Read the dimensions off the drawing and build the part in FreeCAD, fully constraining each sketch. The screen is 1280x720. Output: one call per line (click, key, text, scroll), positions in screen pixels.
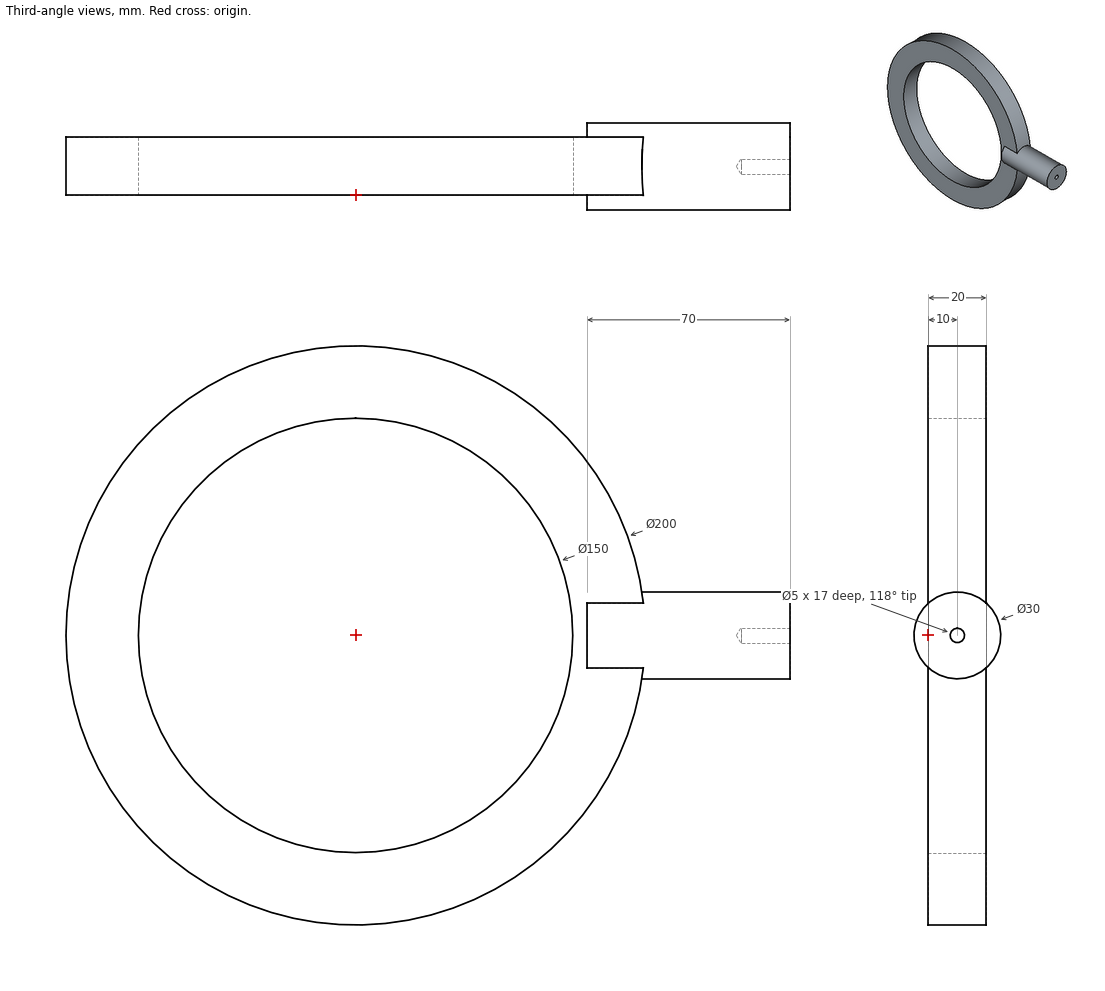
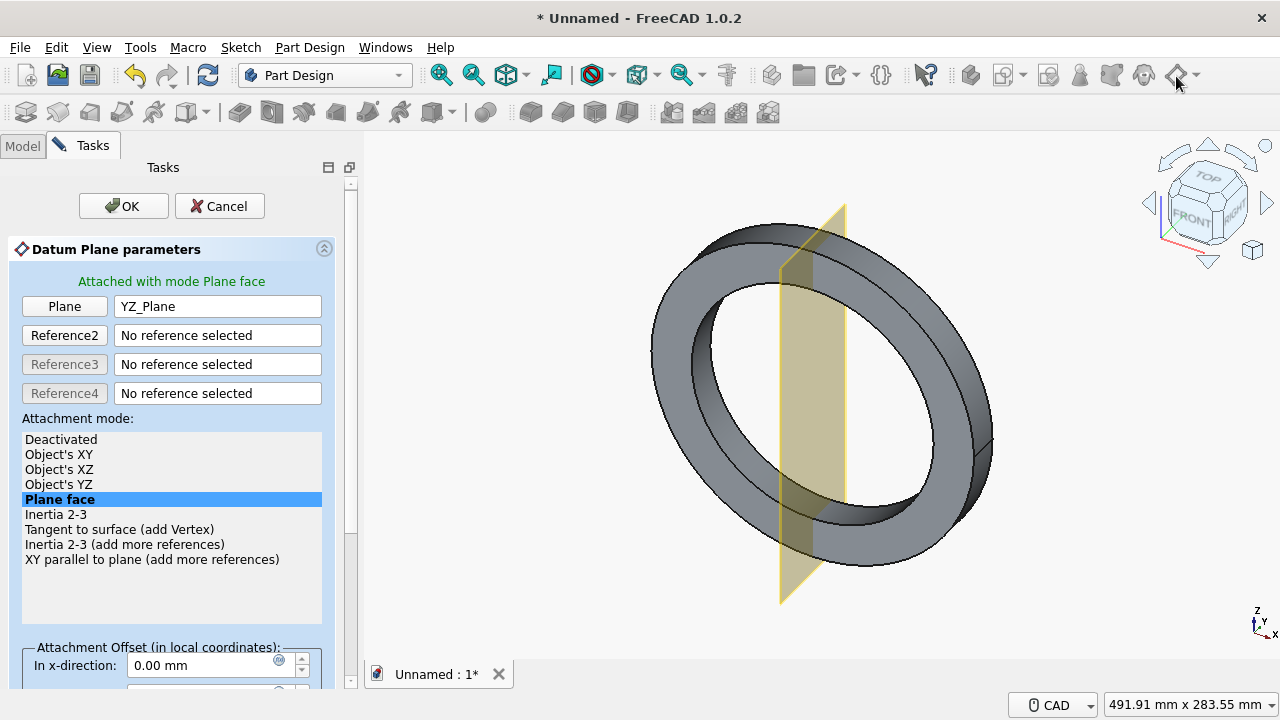
scroll(351, 432, down, 2)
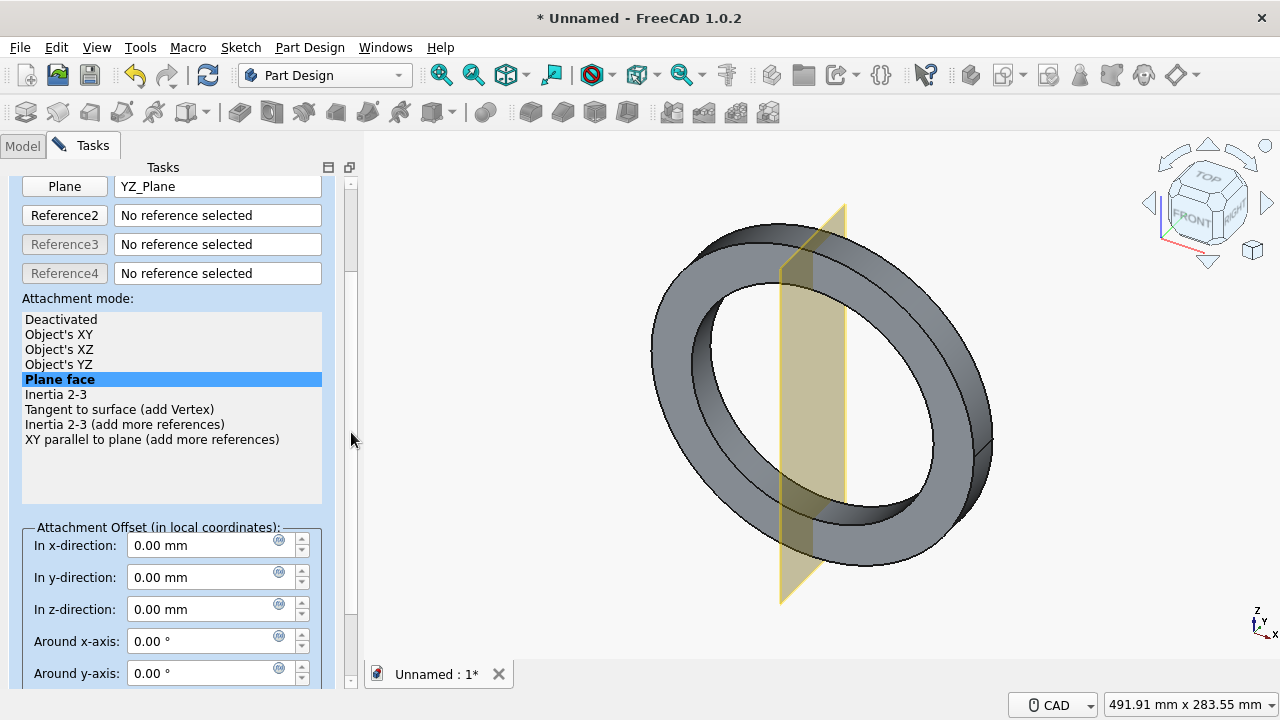
triple_click(210, 609)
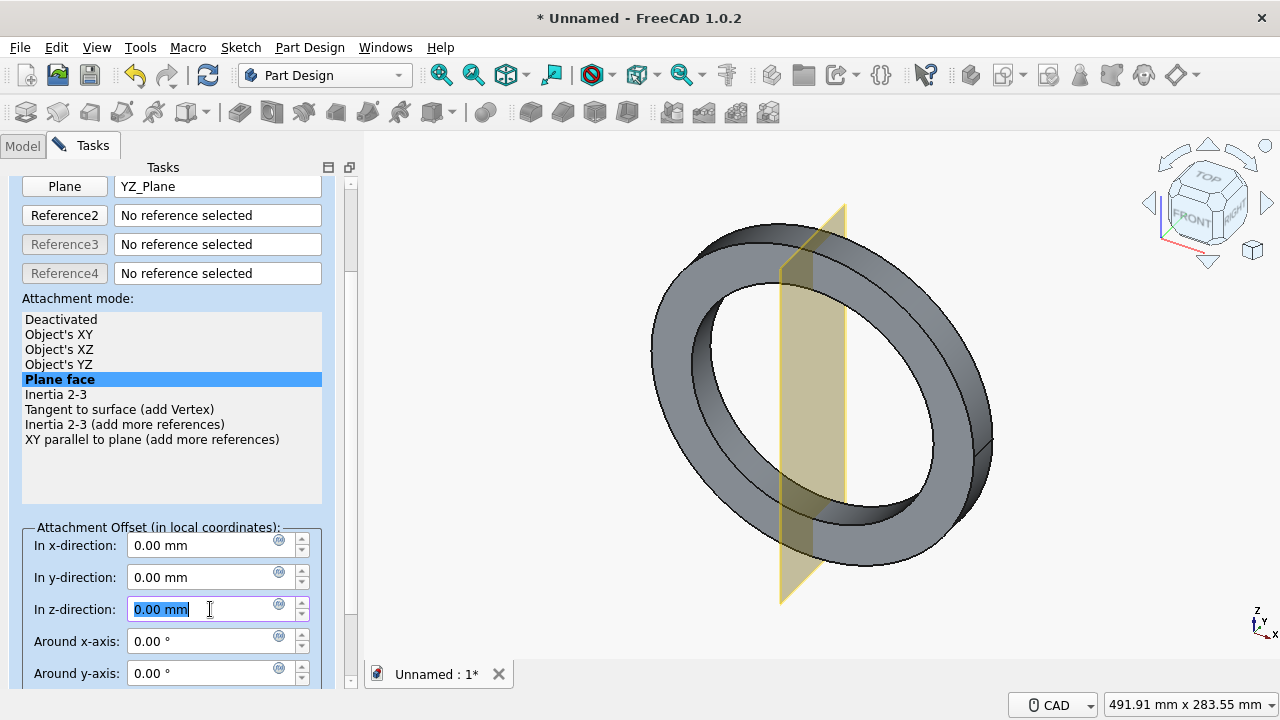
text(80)
key(Tab)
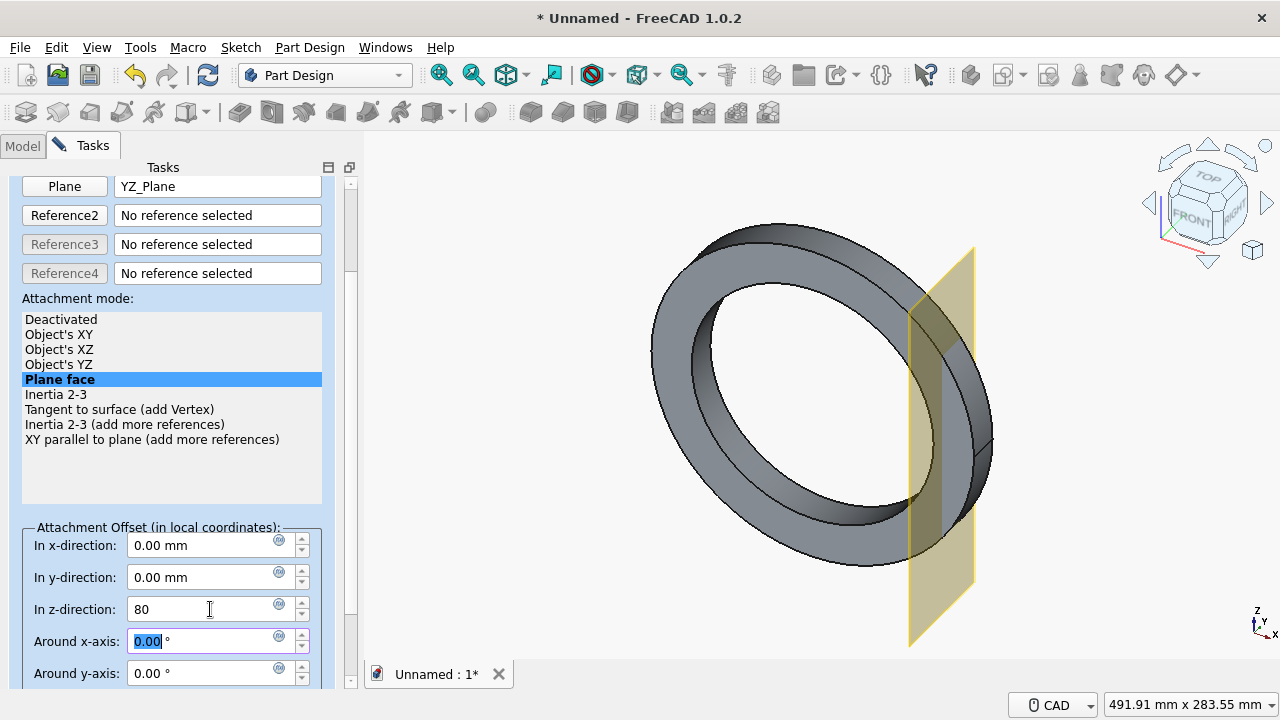
scroll(351, 432, up, 3)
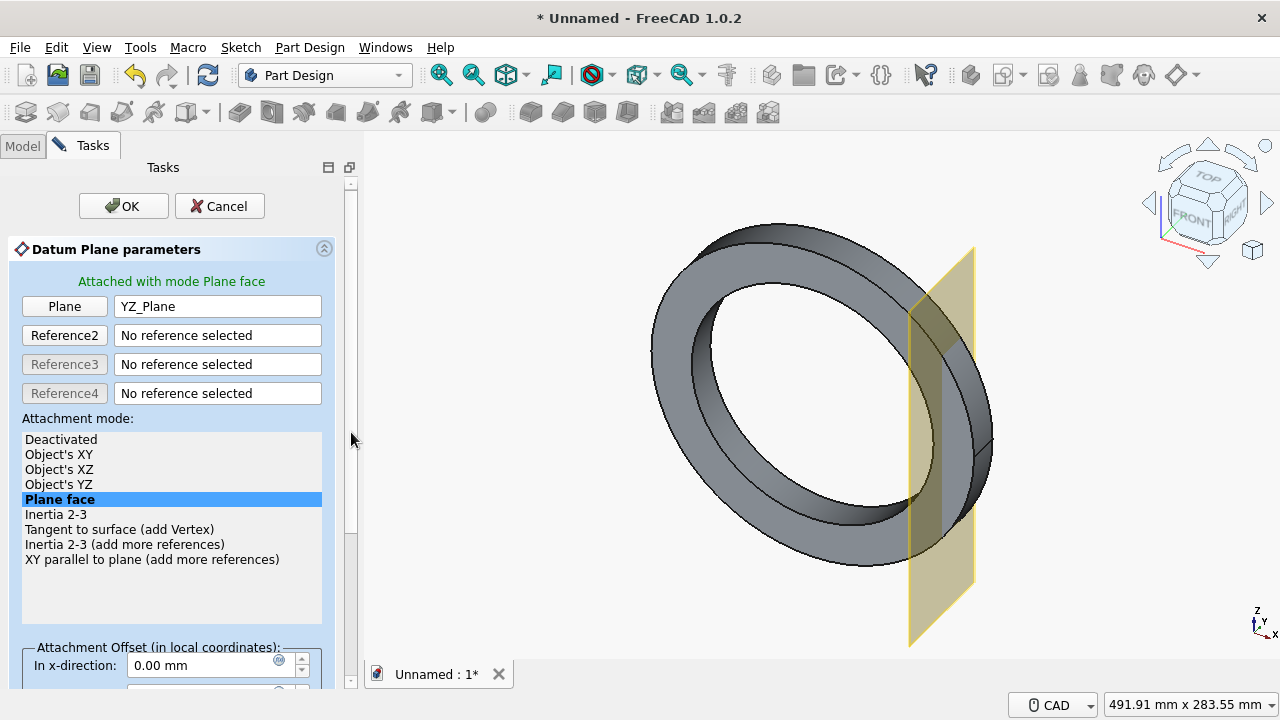
click(124, 206)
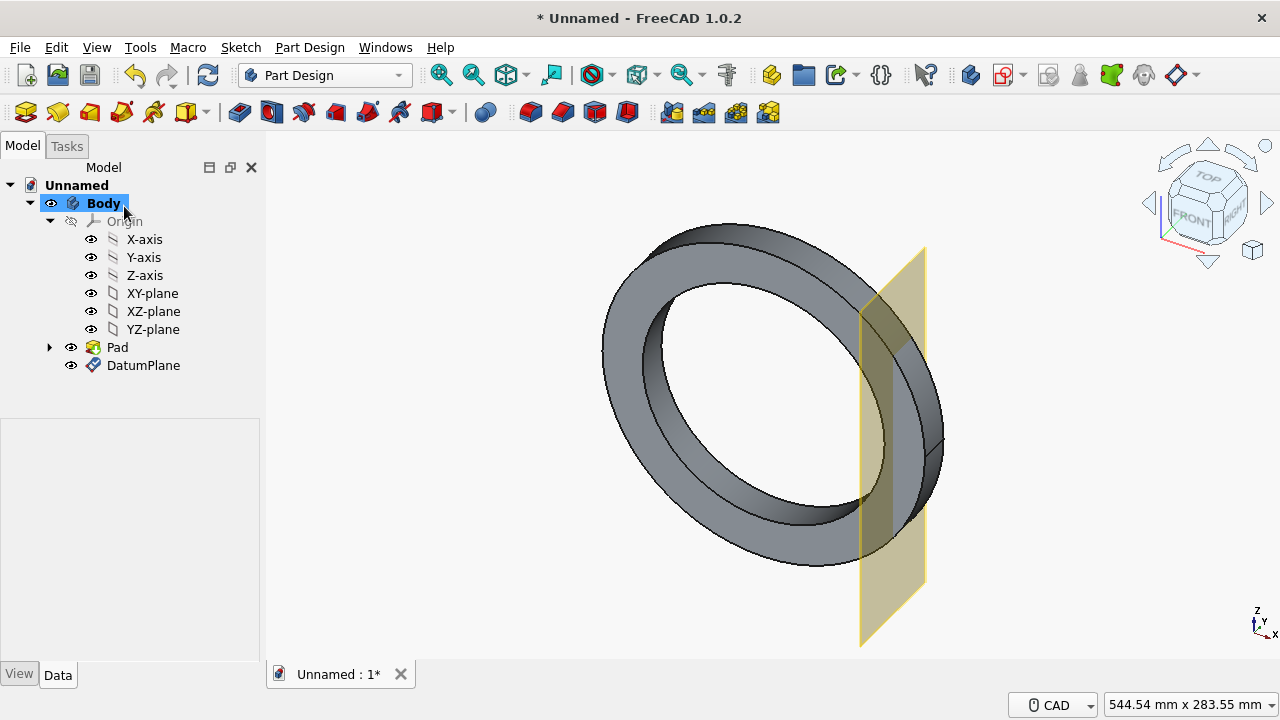
click(116, 365)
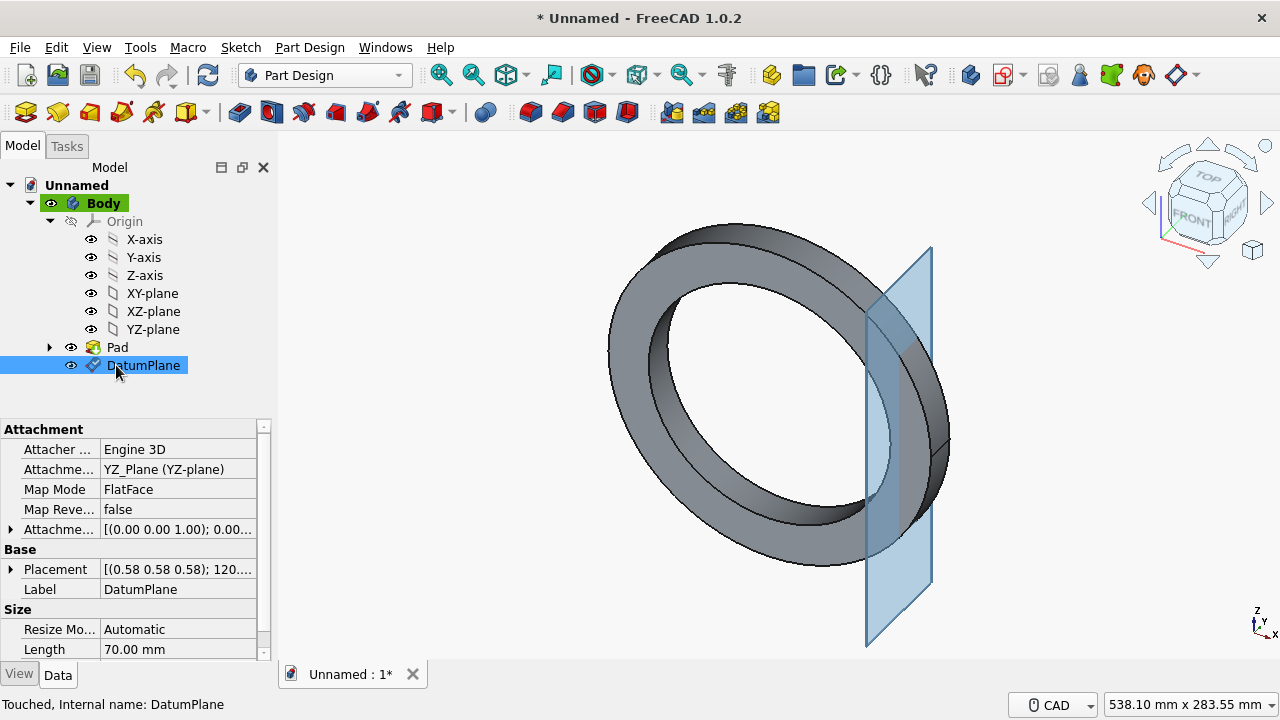
click(1004, 76)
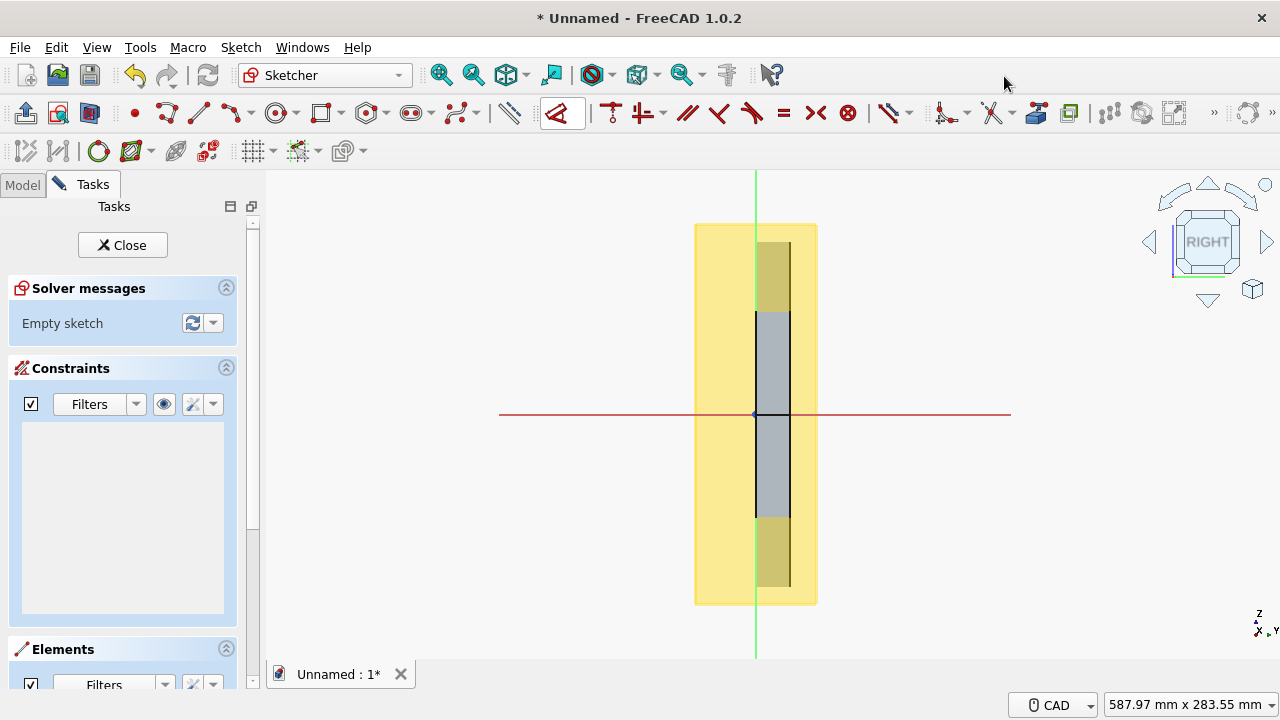
key(q)
key(s)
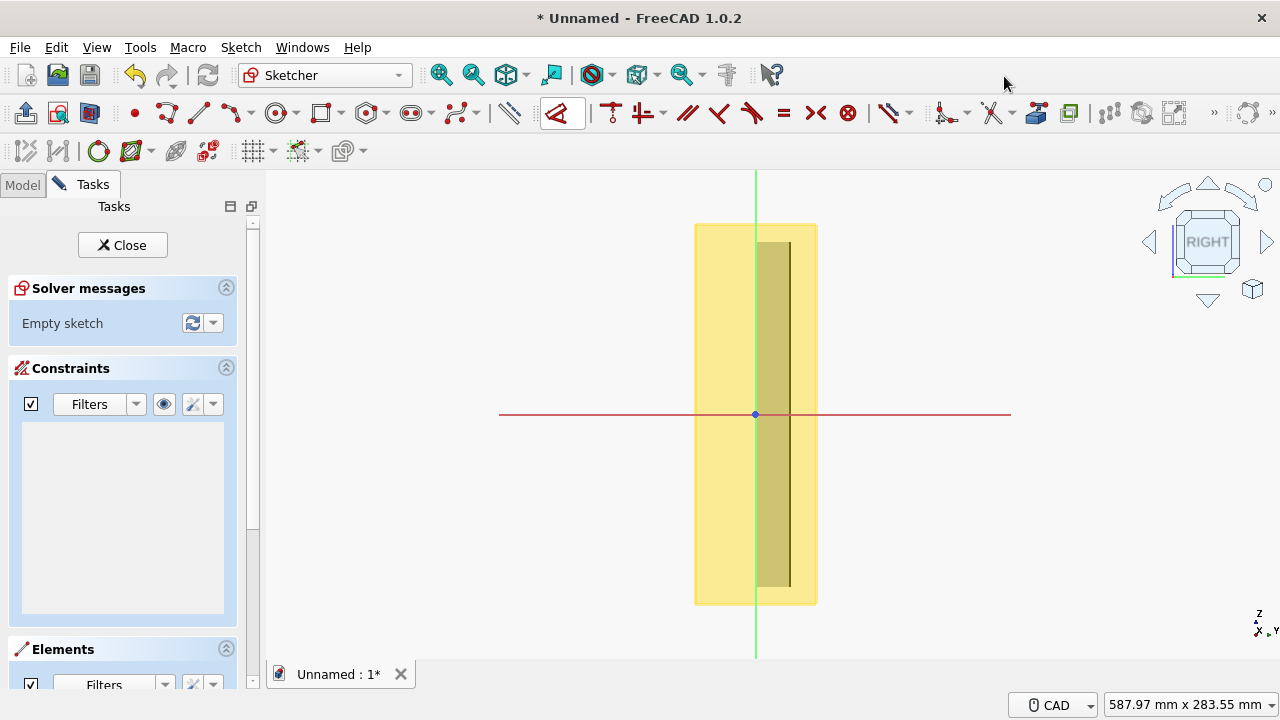
scroll(787, 414, up, 9)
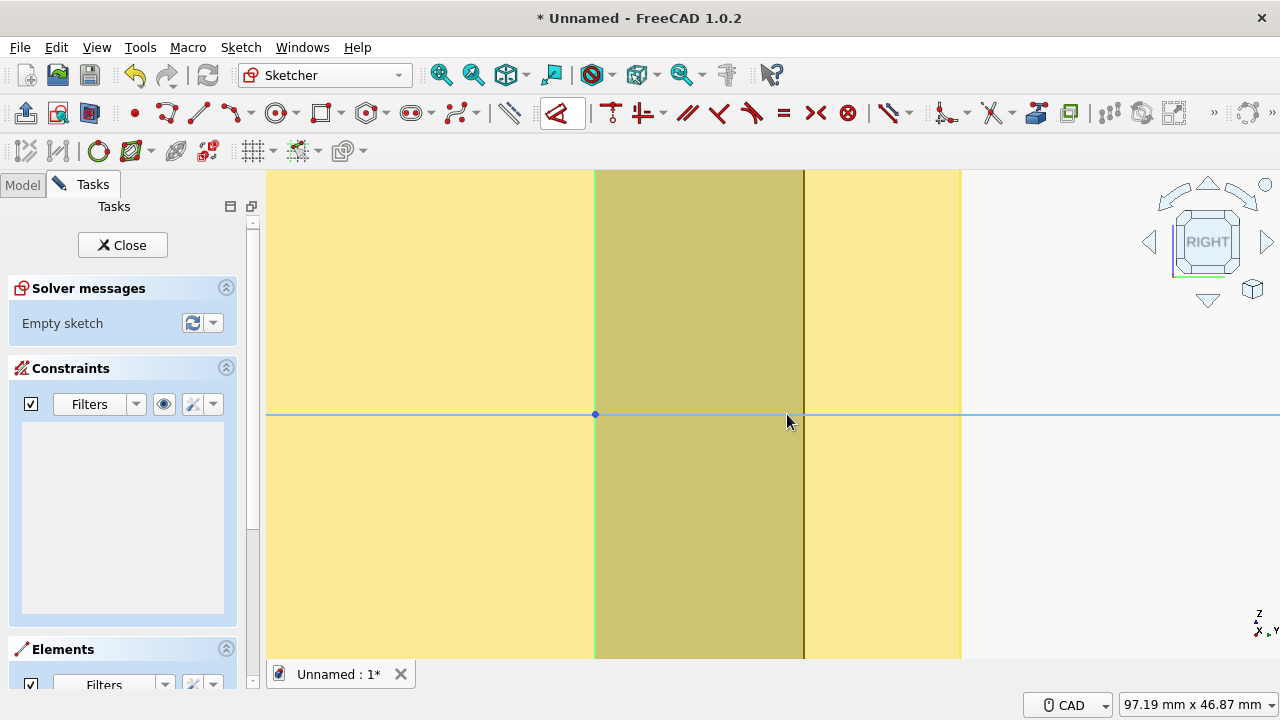
key(g)
key(c)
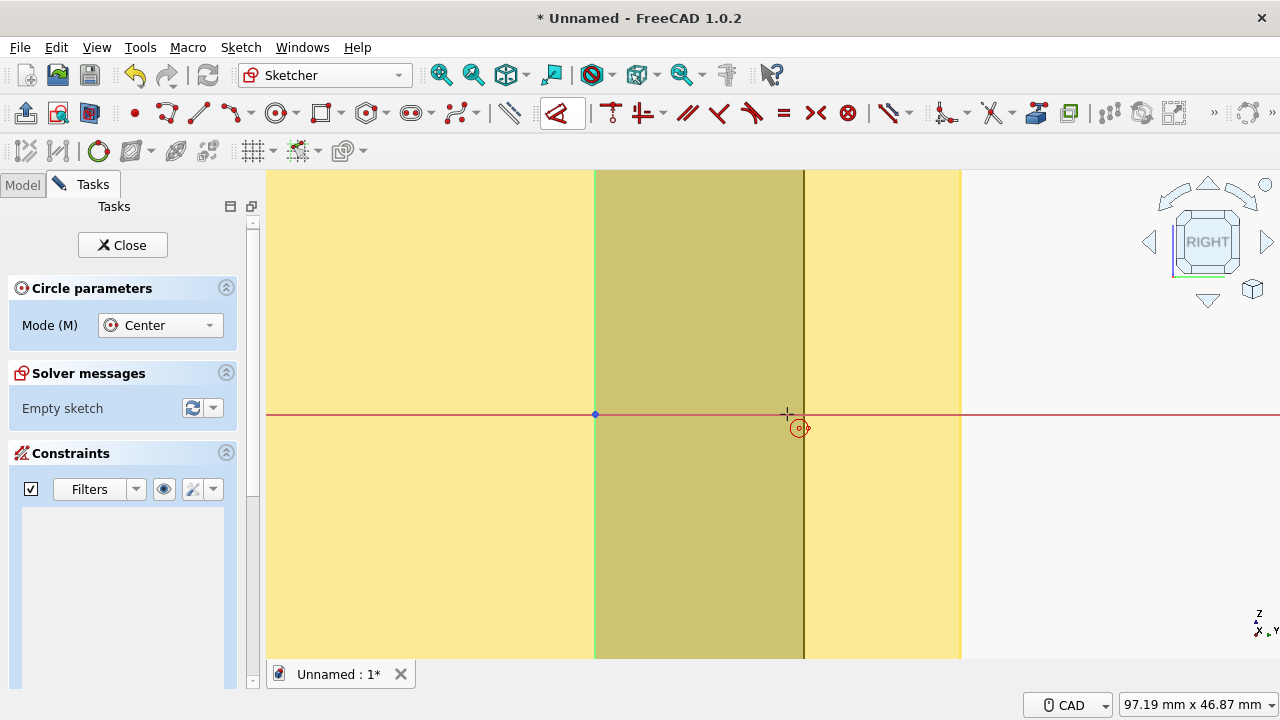
click(700, 414)
click(810, 304)
key(Escape)